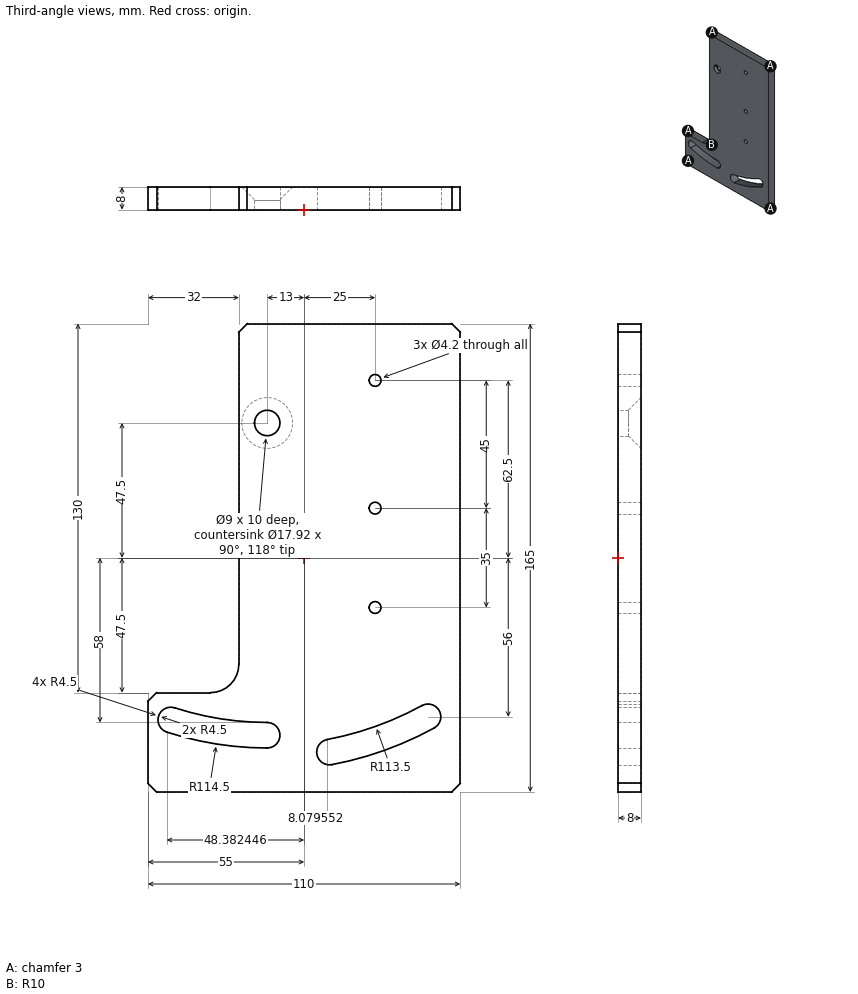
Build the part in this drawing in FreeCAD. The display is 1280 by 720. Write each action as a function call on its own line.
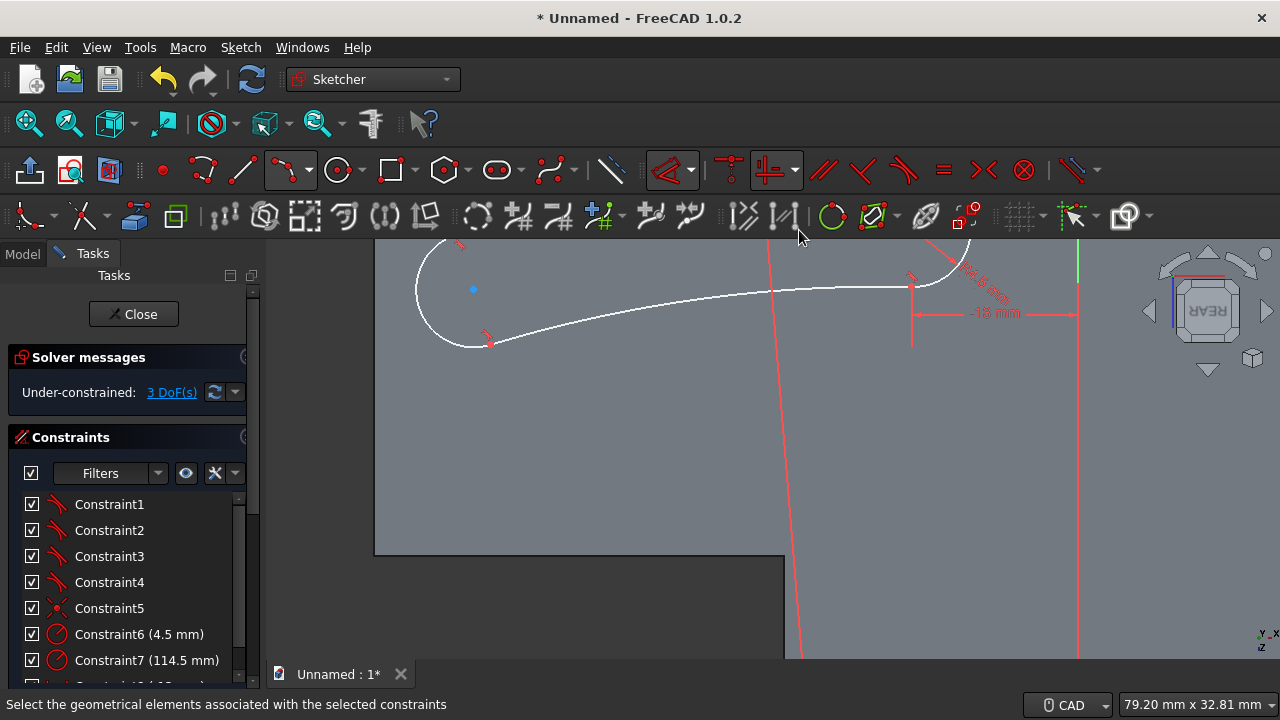
click(912, 287)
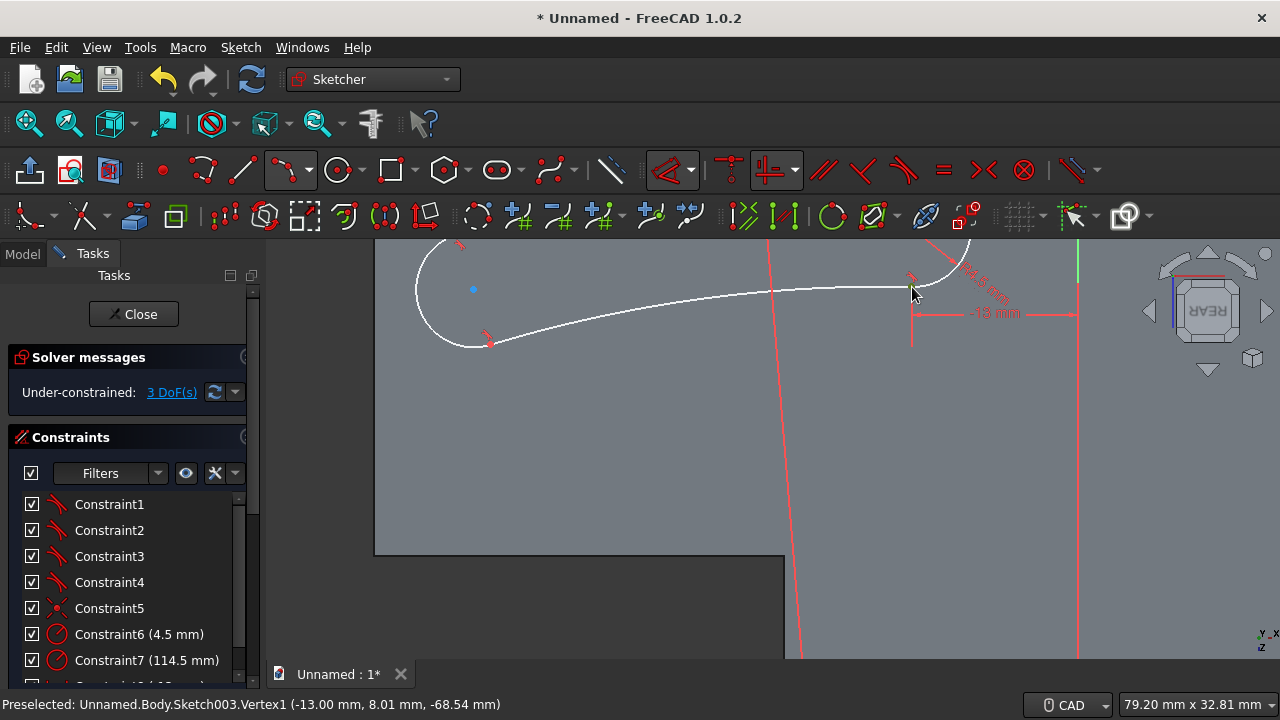
click(694, 170)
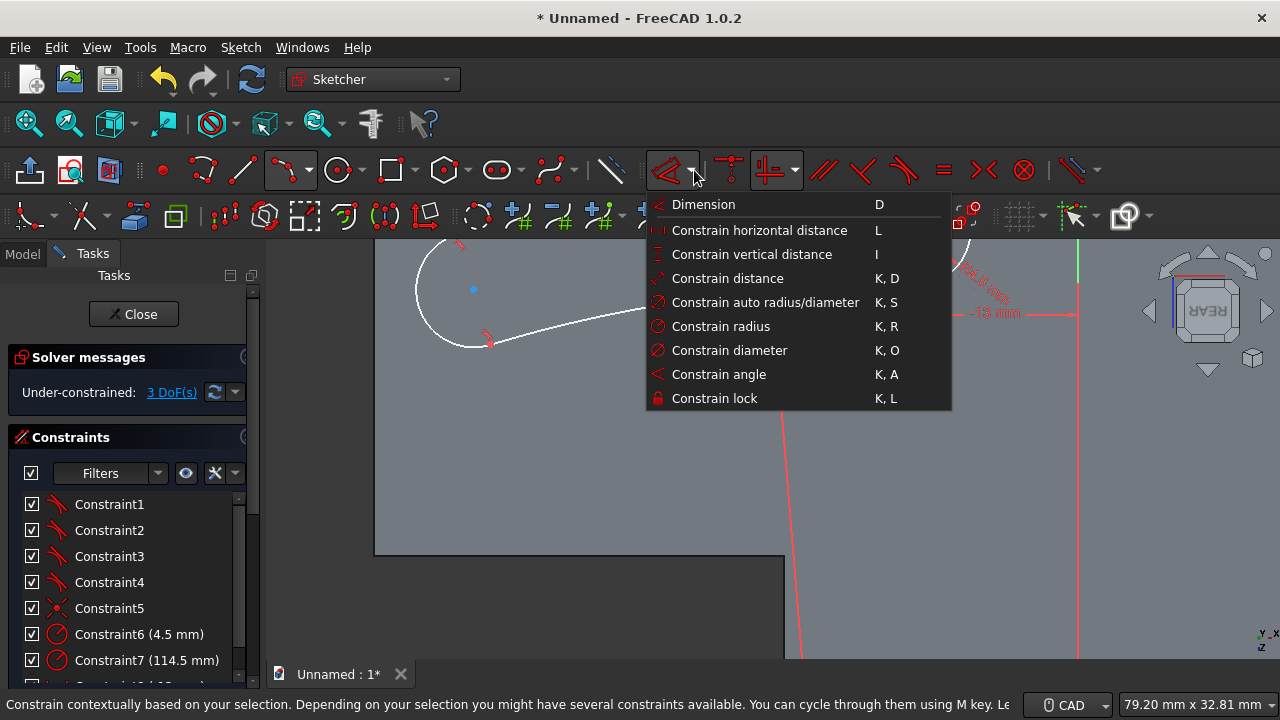
click(799, 254)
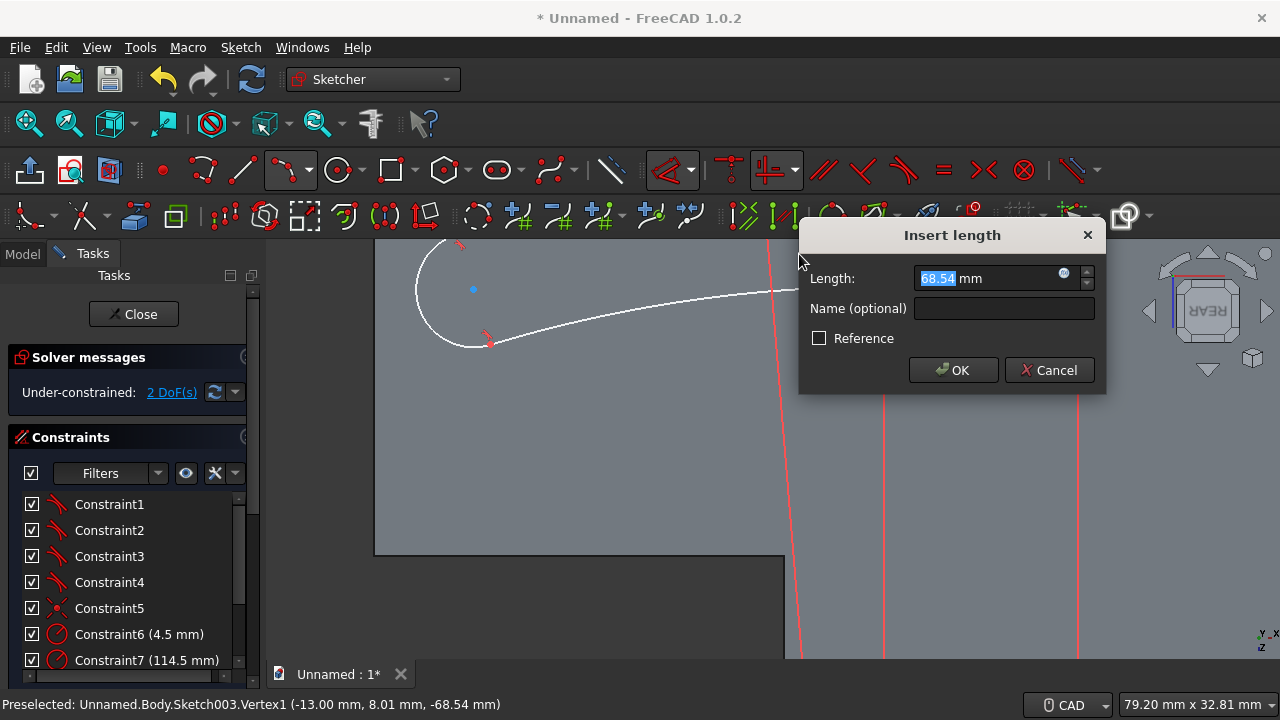
text(58)
key(Return)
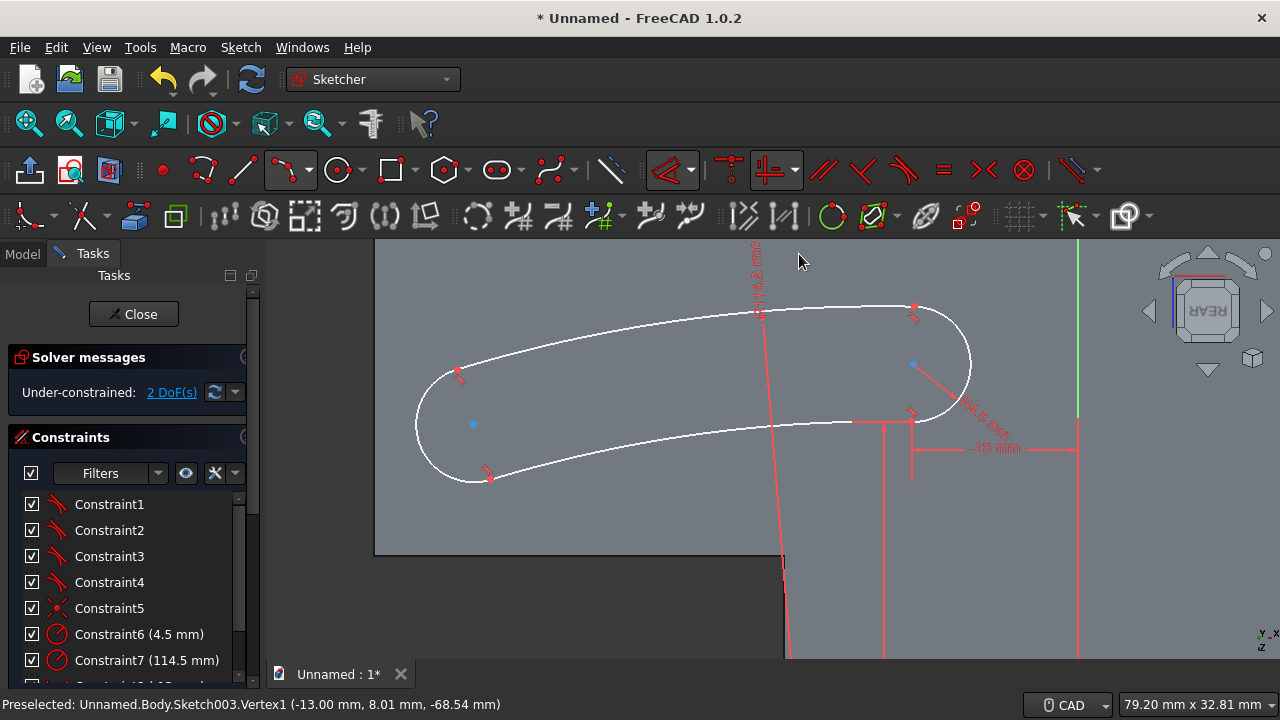
scroll(685, 326, down, 6)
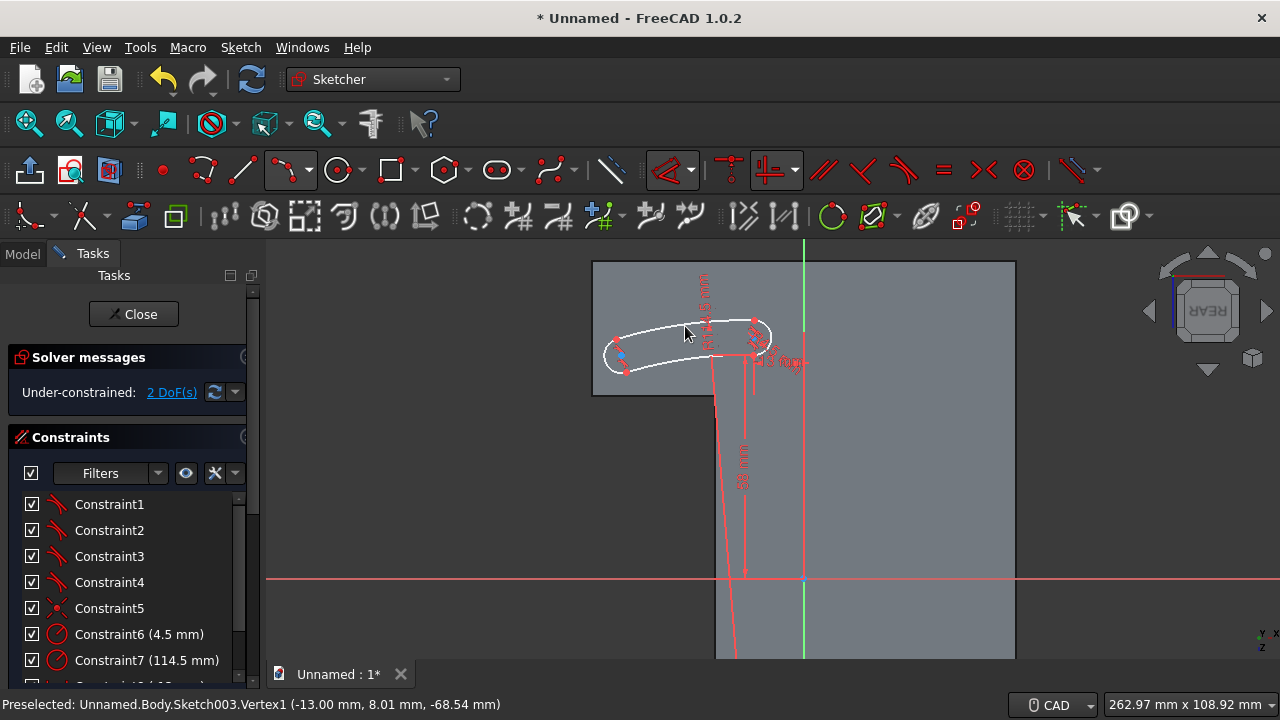
scroll(704, 337, down, 3)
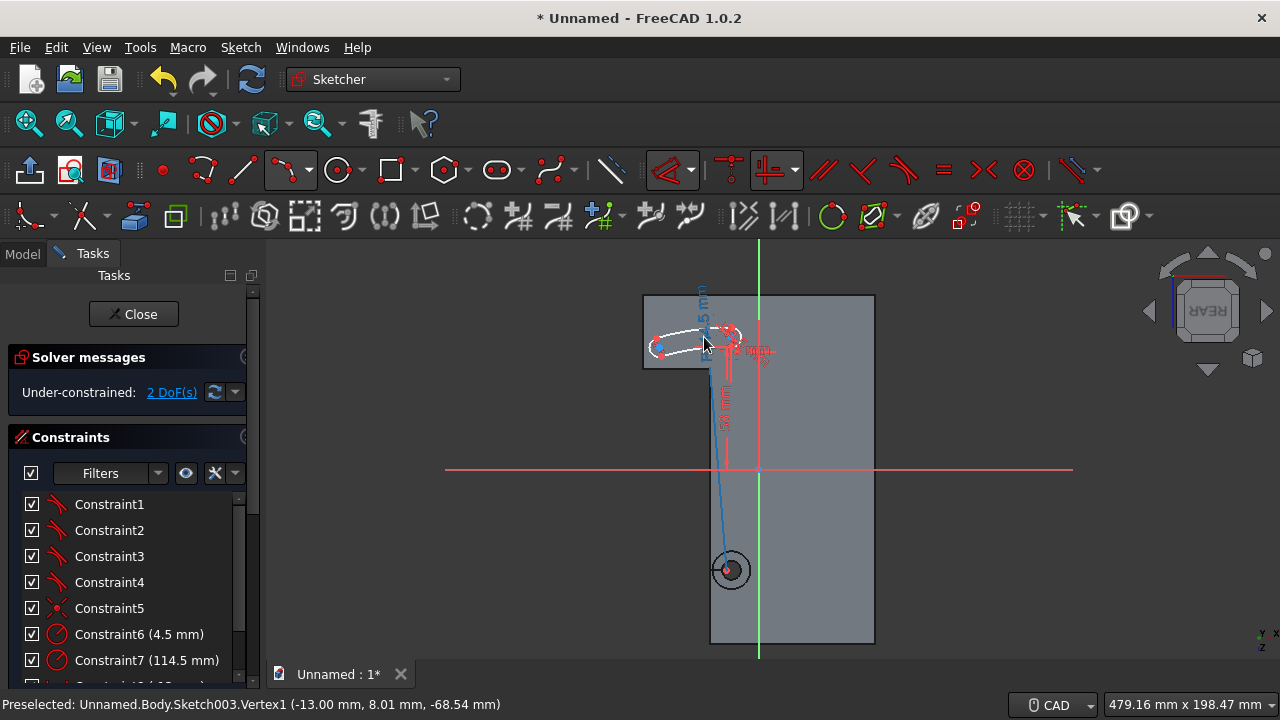
scroll(727, 570, up, 2)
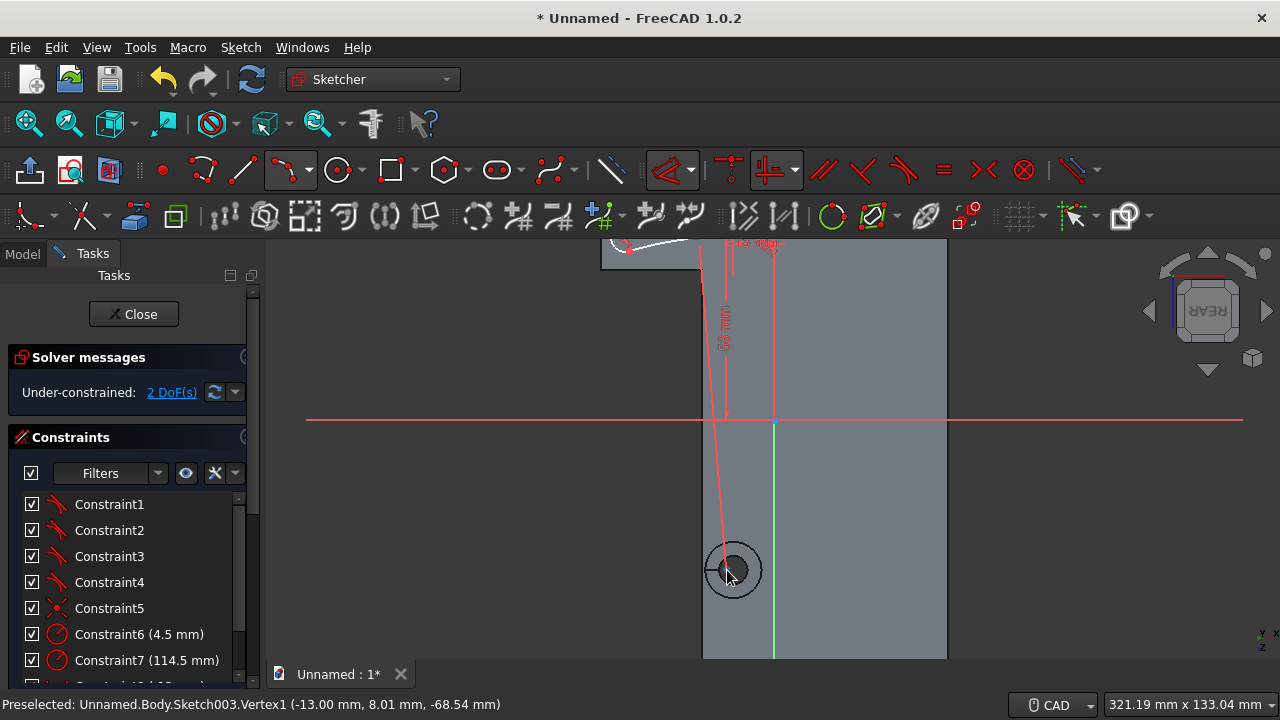
click(726, 570)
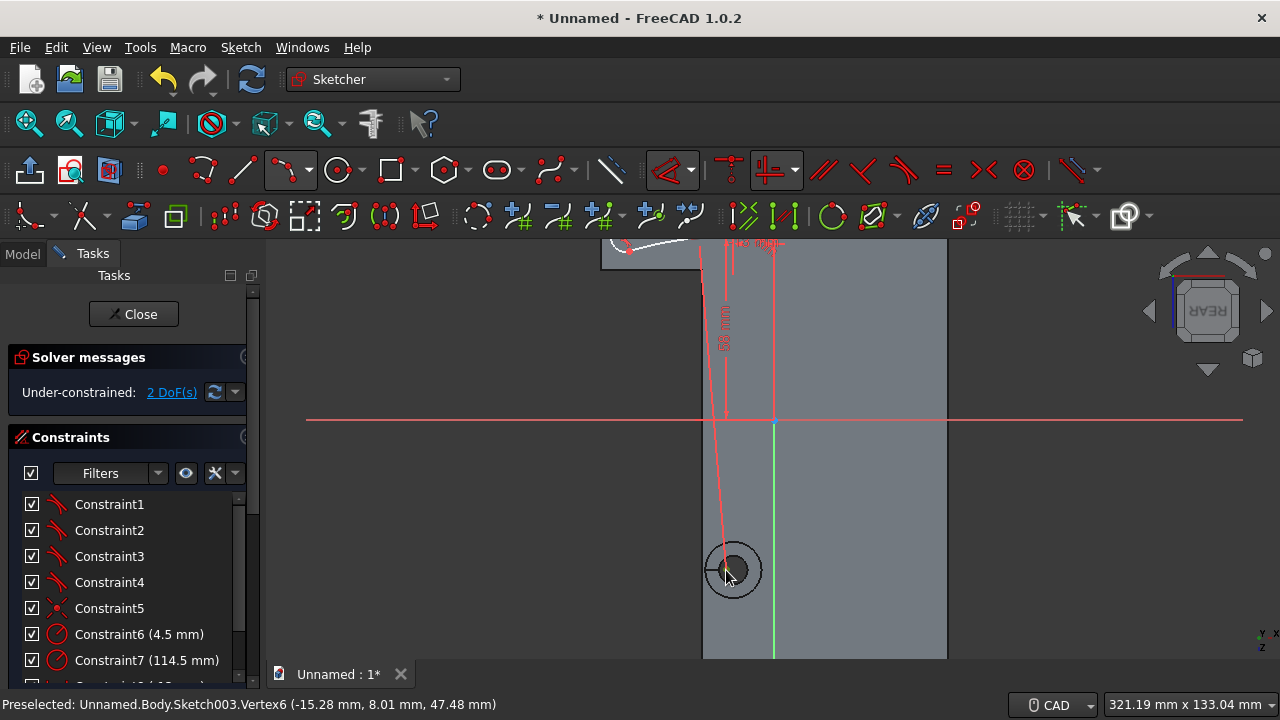
key(l)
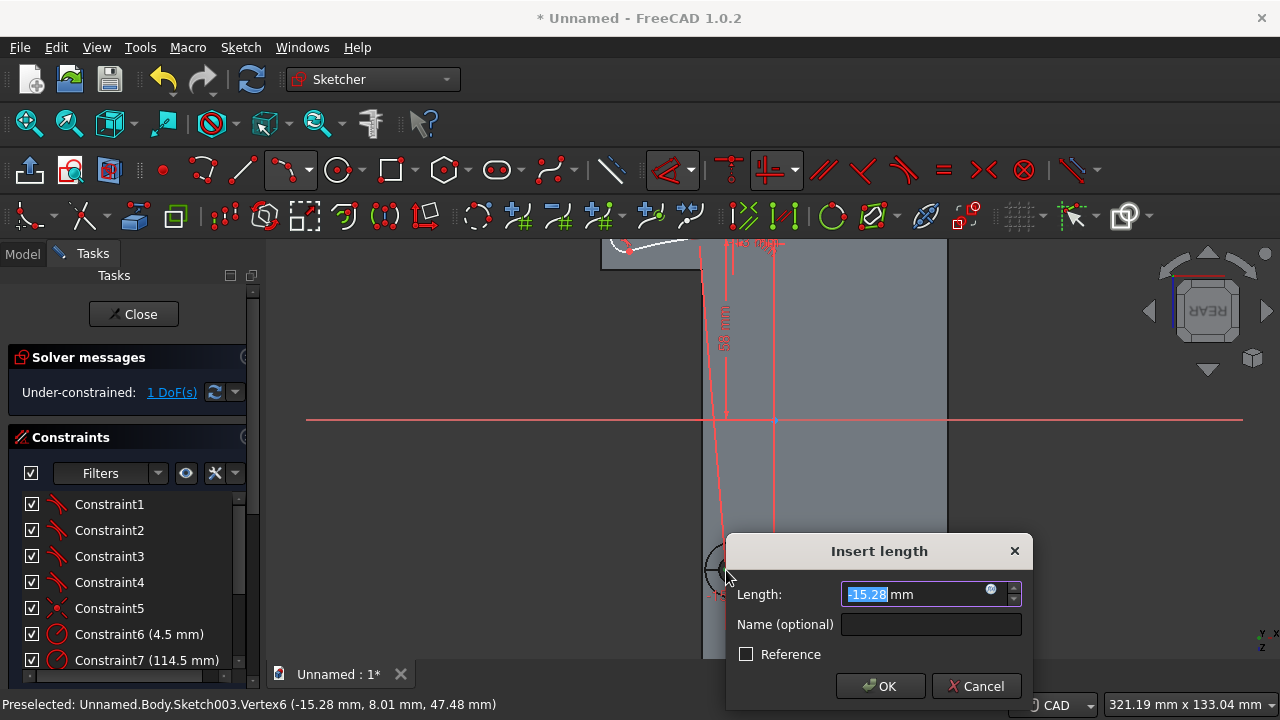
text(-13)
key(Return)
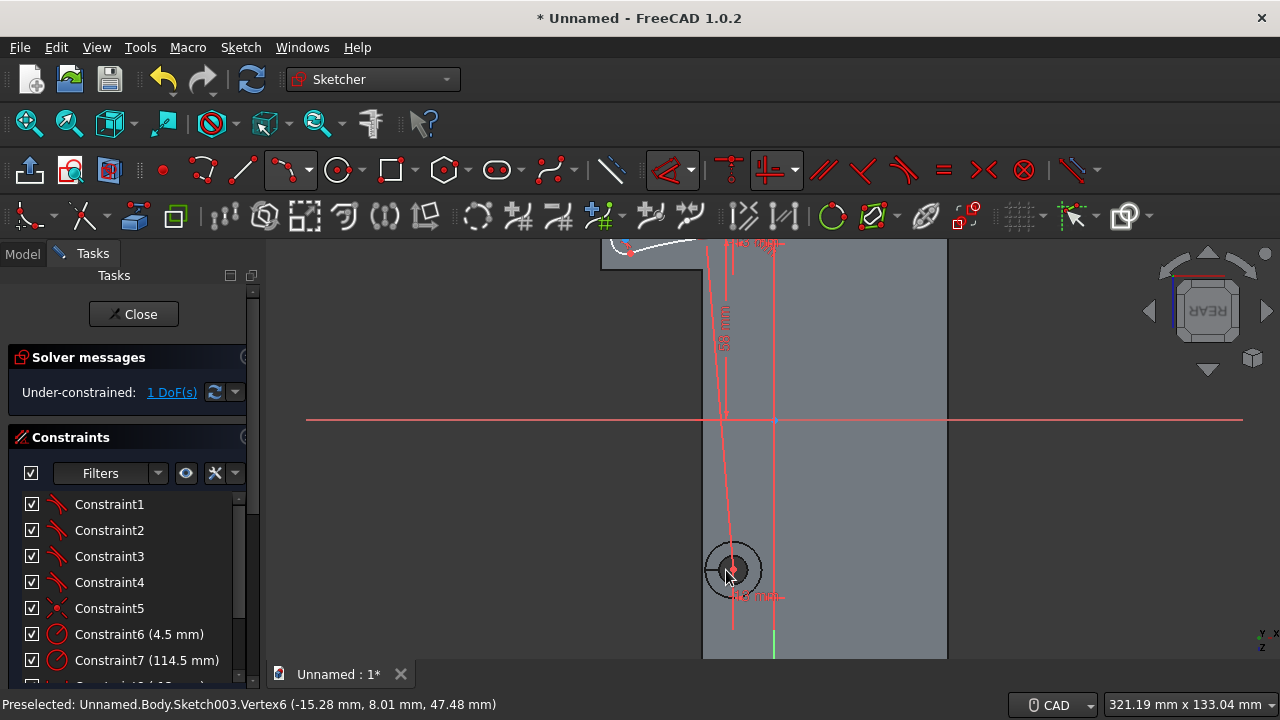
scroll(727, 631, down, 2)